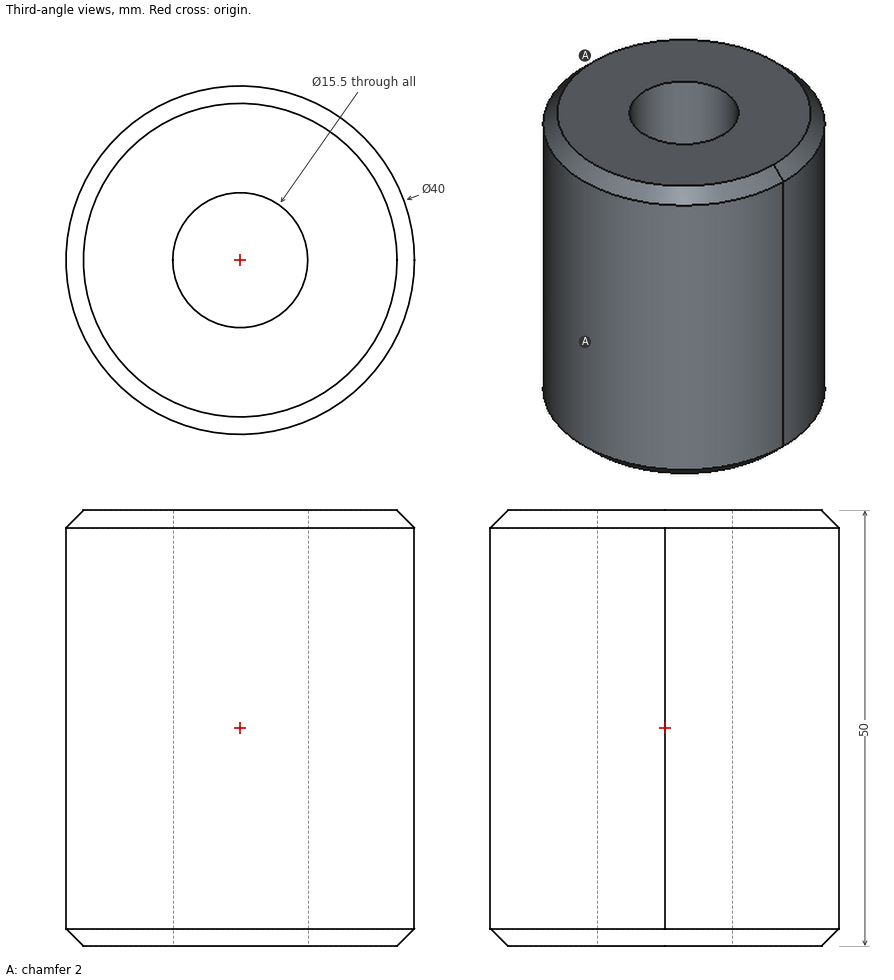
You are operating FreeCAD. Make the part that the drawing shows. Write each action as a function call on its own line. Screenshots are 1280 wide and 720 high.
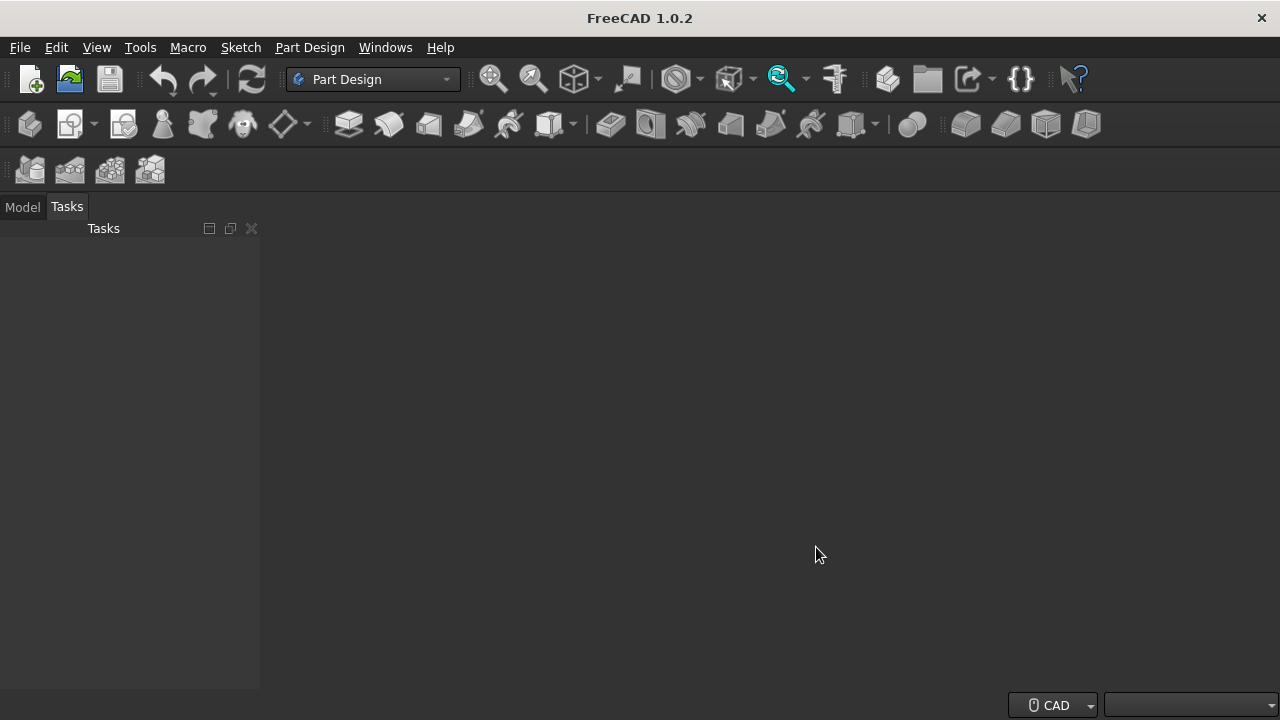
key(ctrl+n)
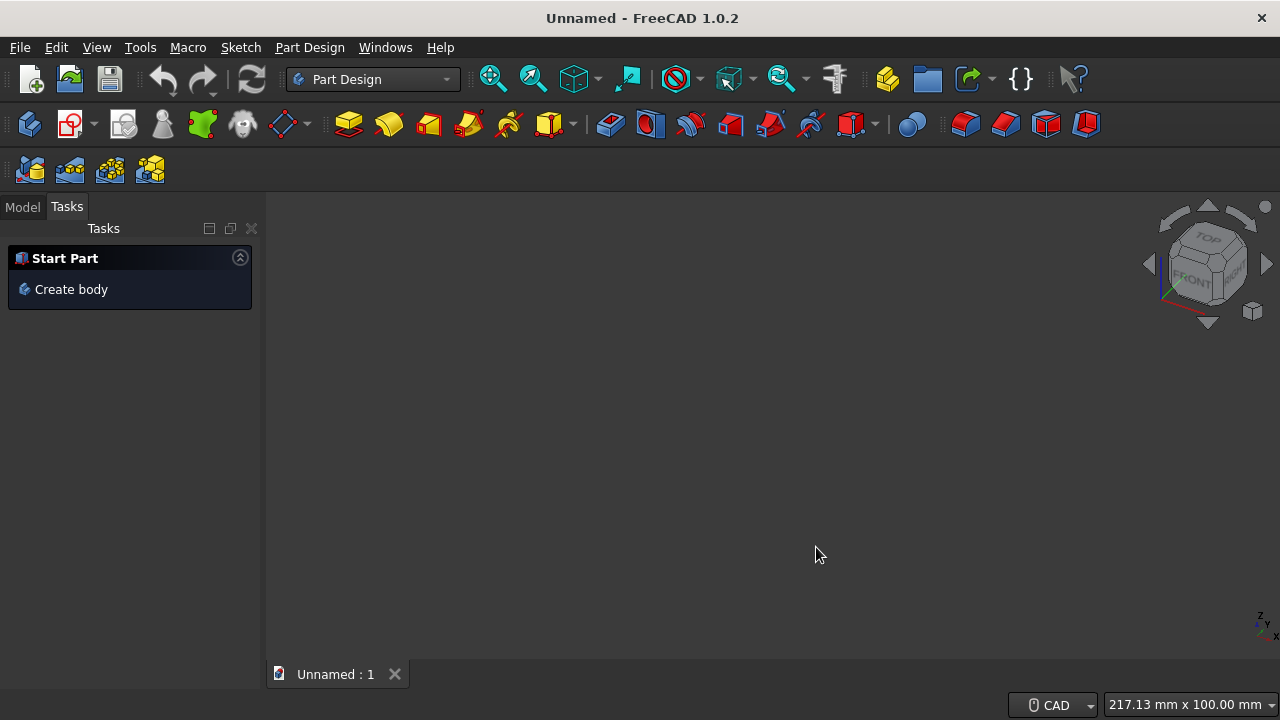
click(70, 124)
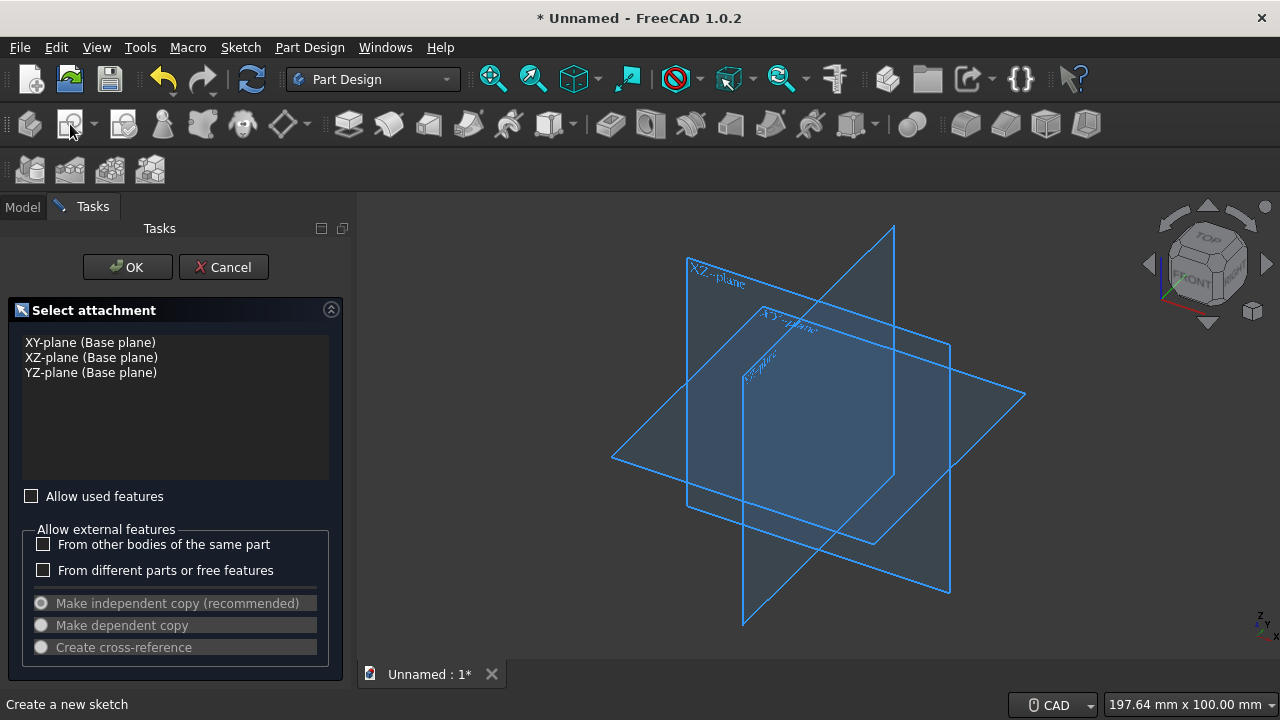
click(82, 342)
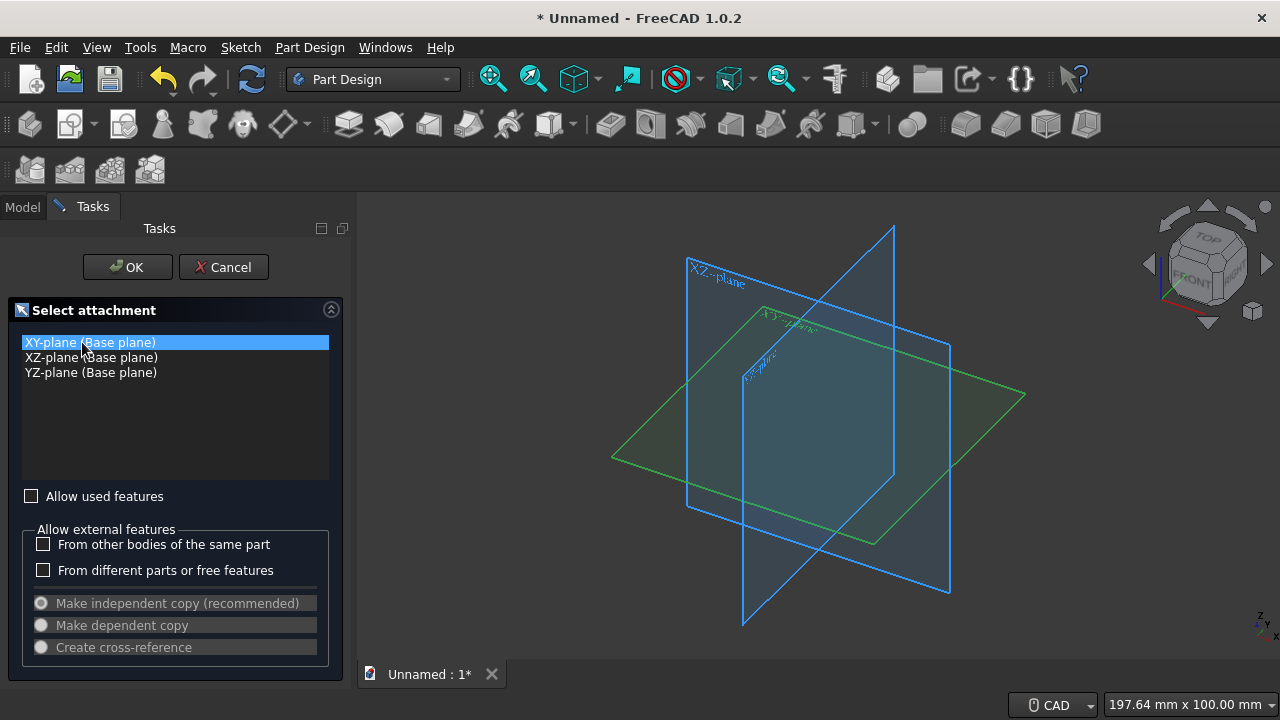
click(128, 267)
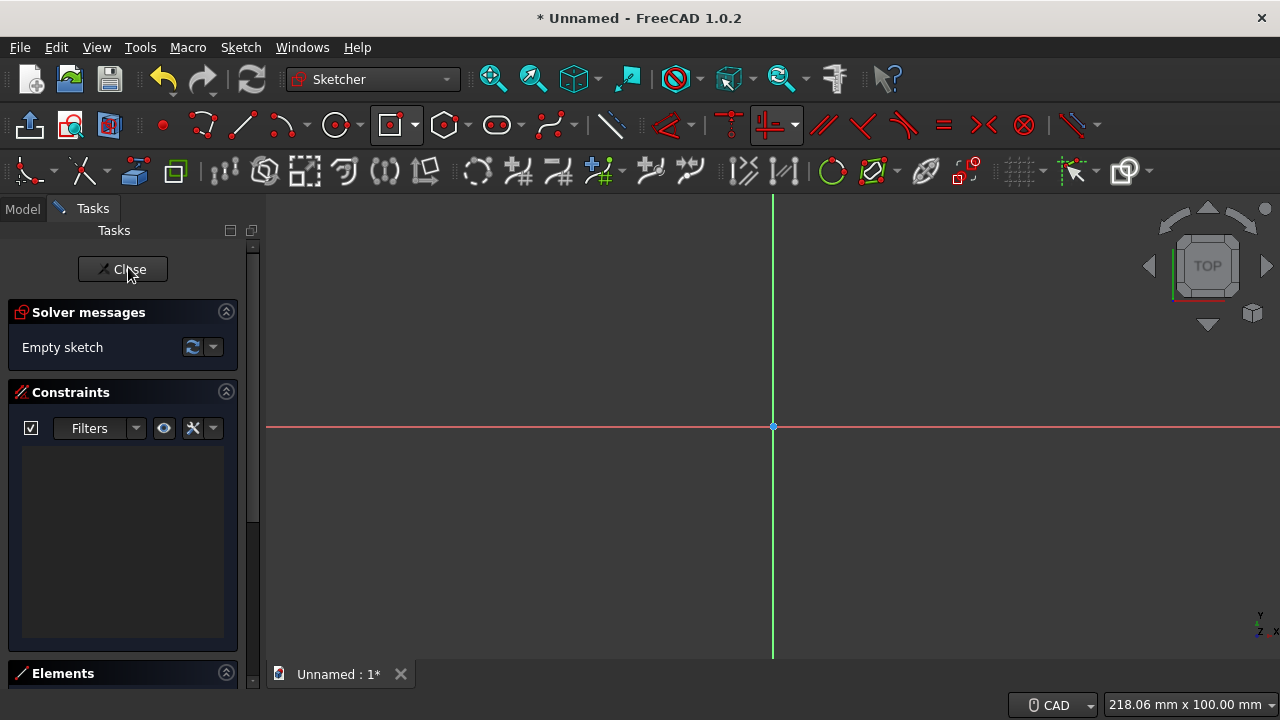
scroll(912, 426, up, 2)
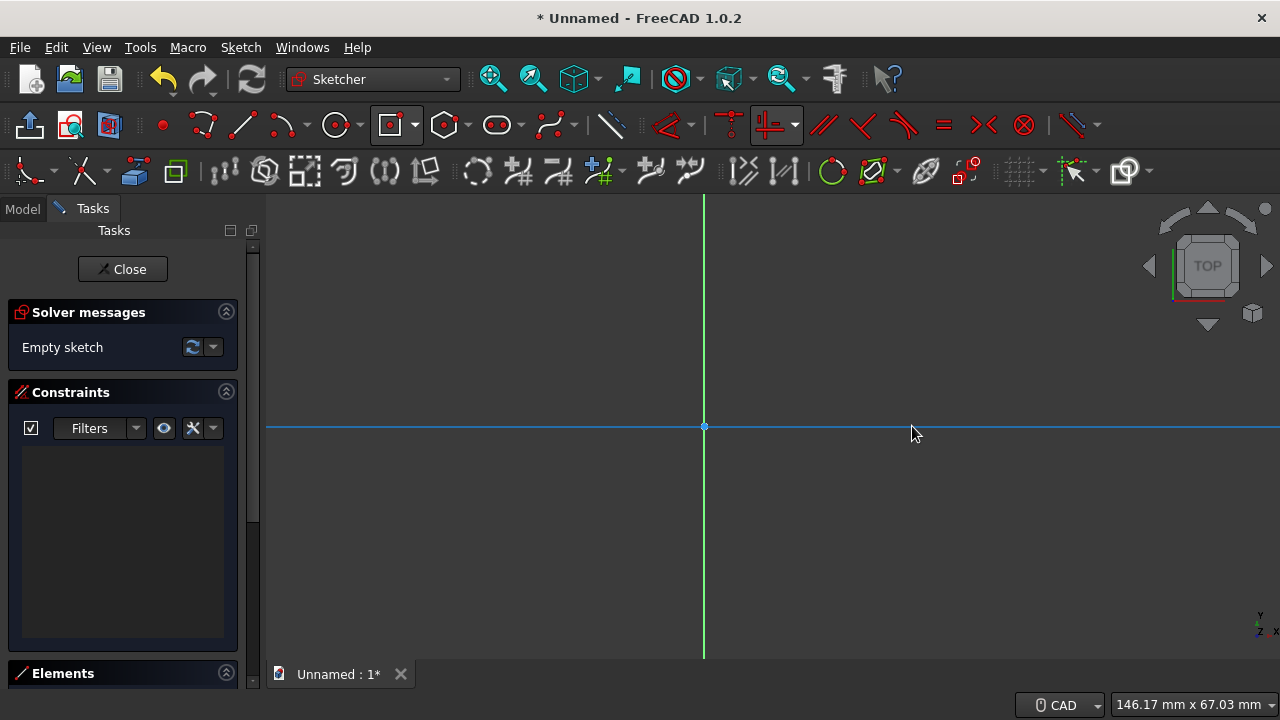
key(g)
key(c)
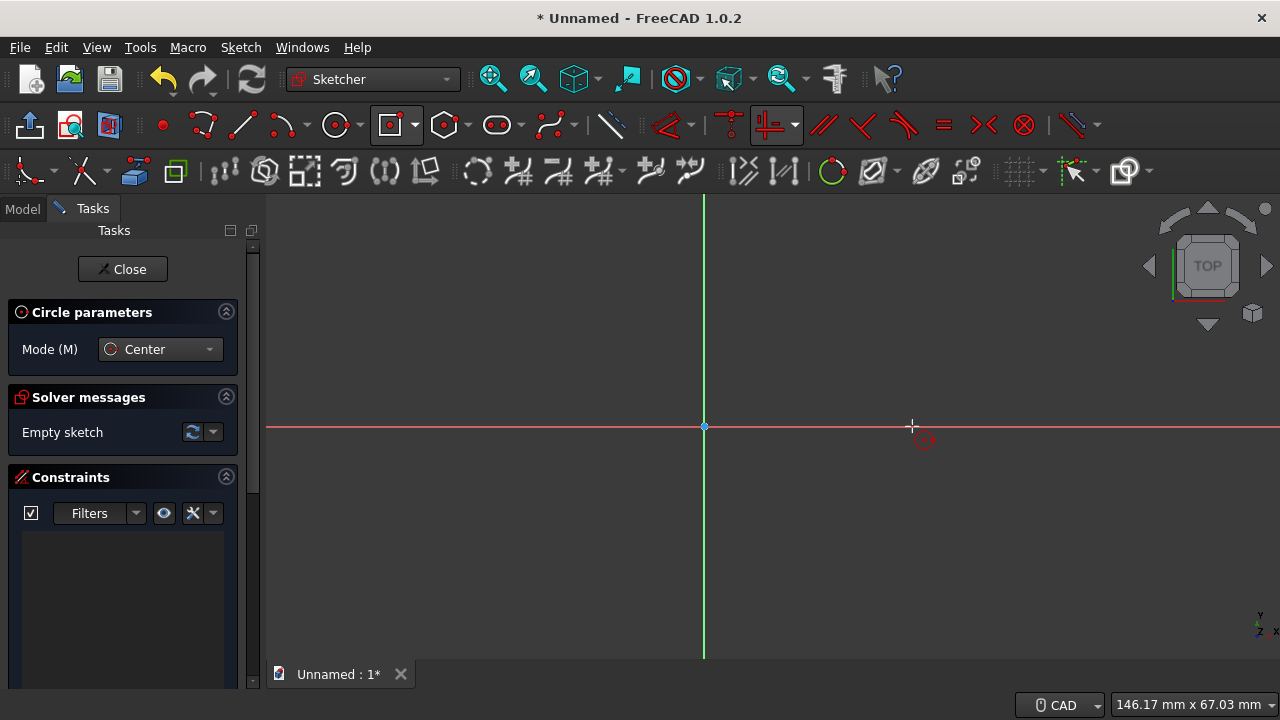
click(704, 426)
move(802, 328)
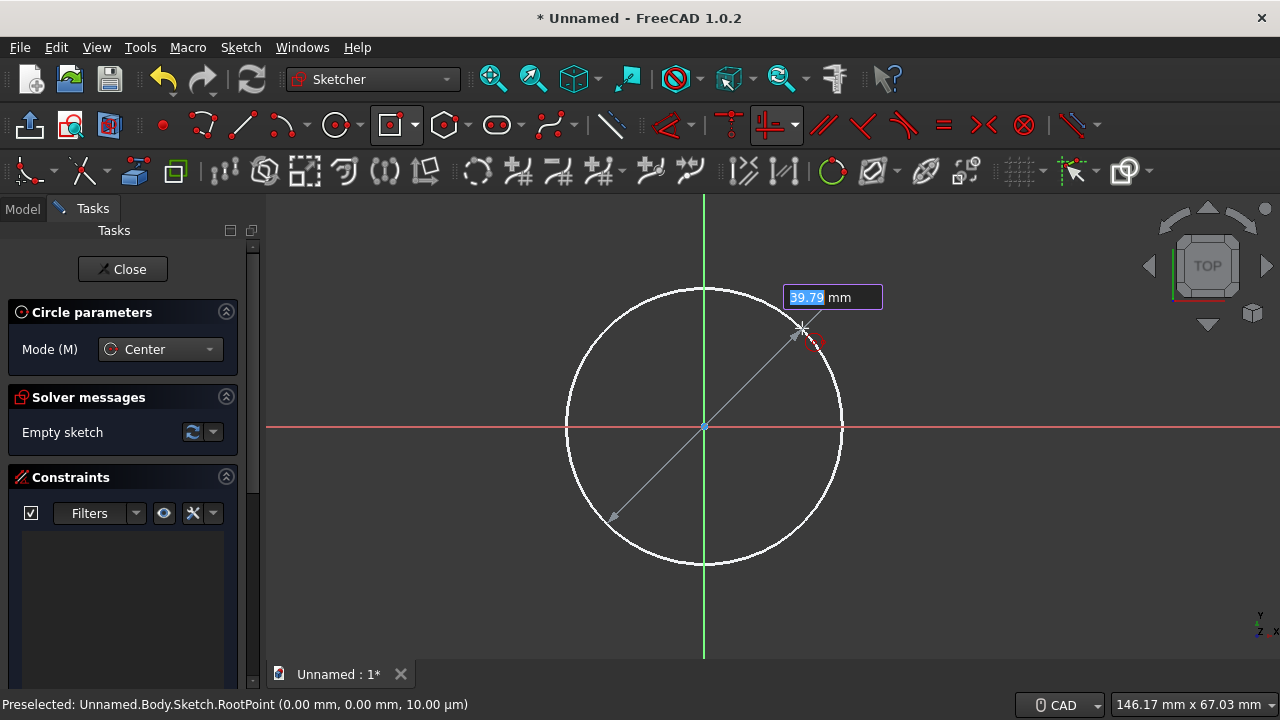
text(40)
key(Return)
key(Escape)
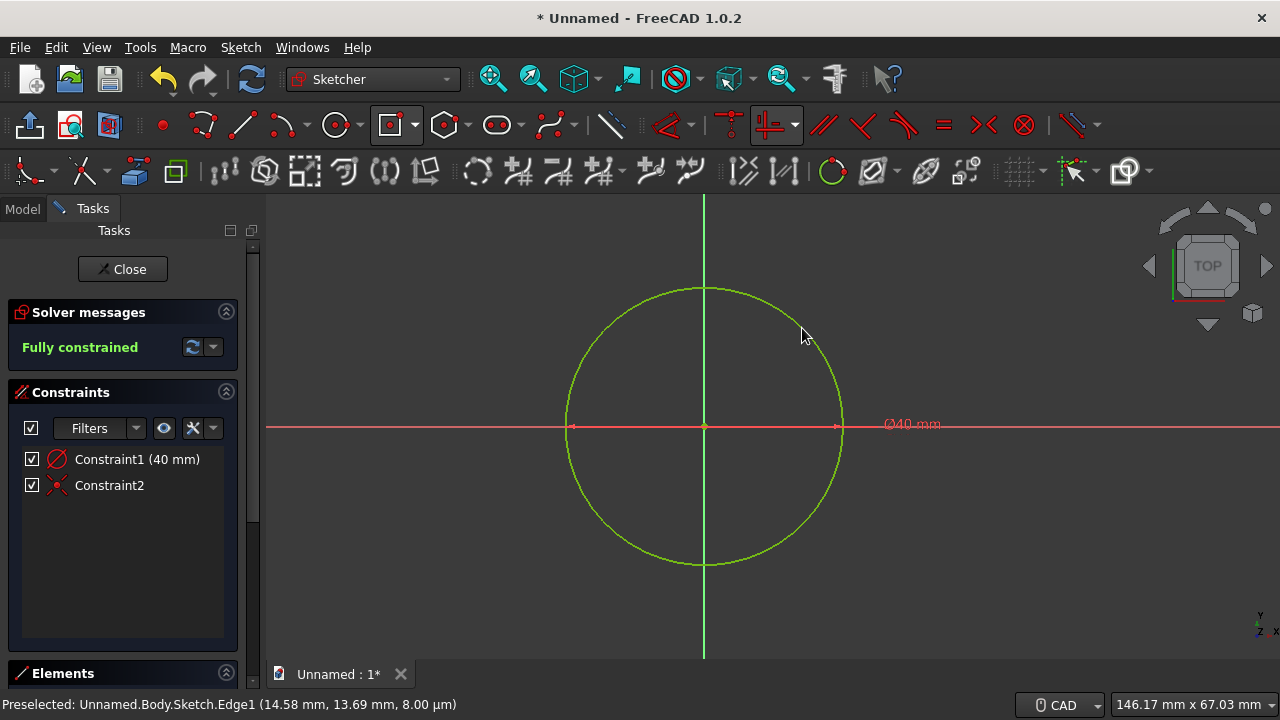
click(123, 269)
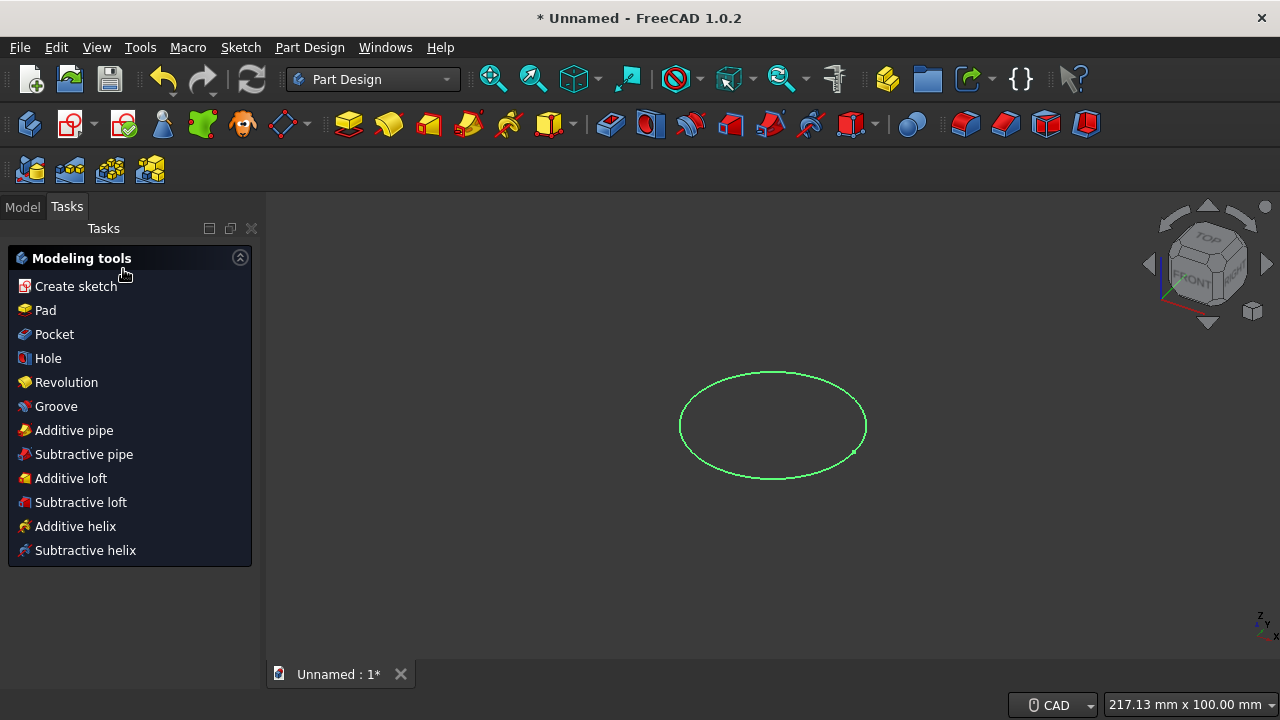
click(350, 124)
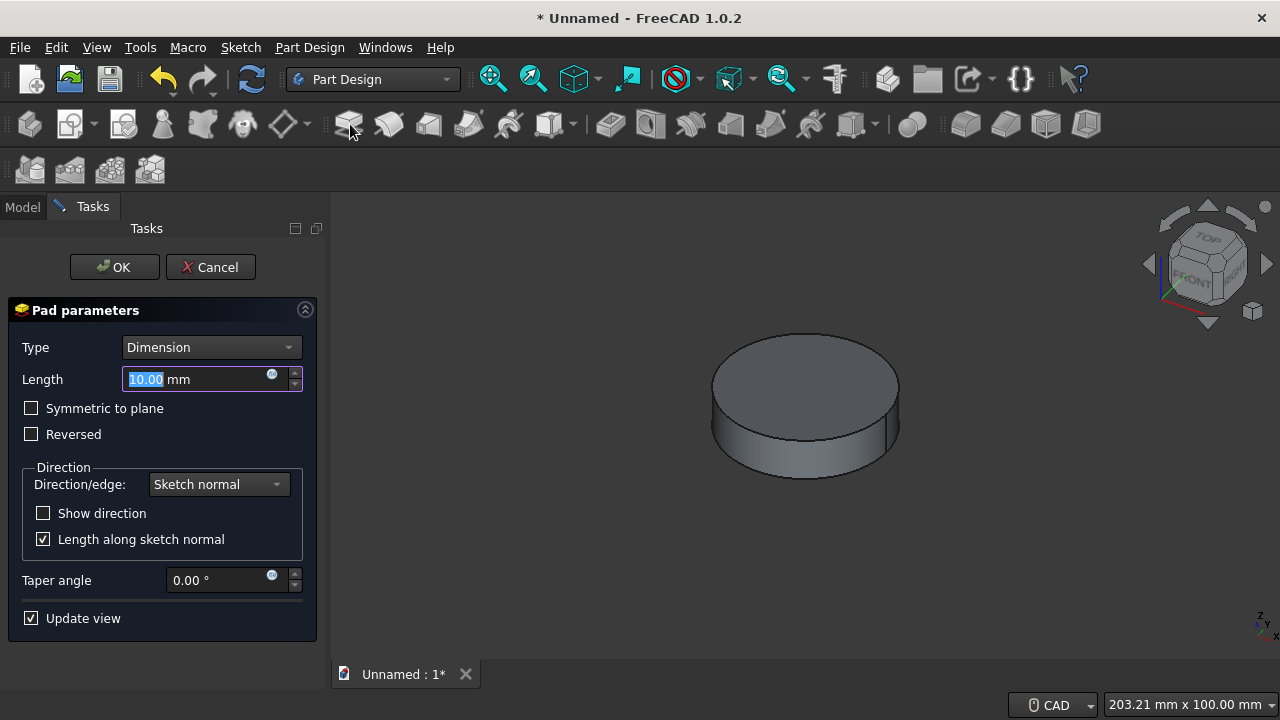
text(50)
key(Tab)